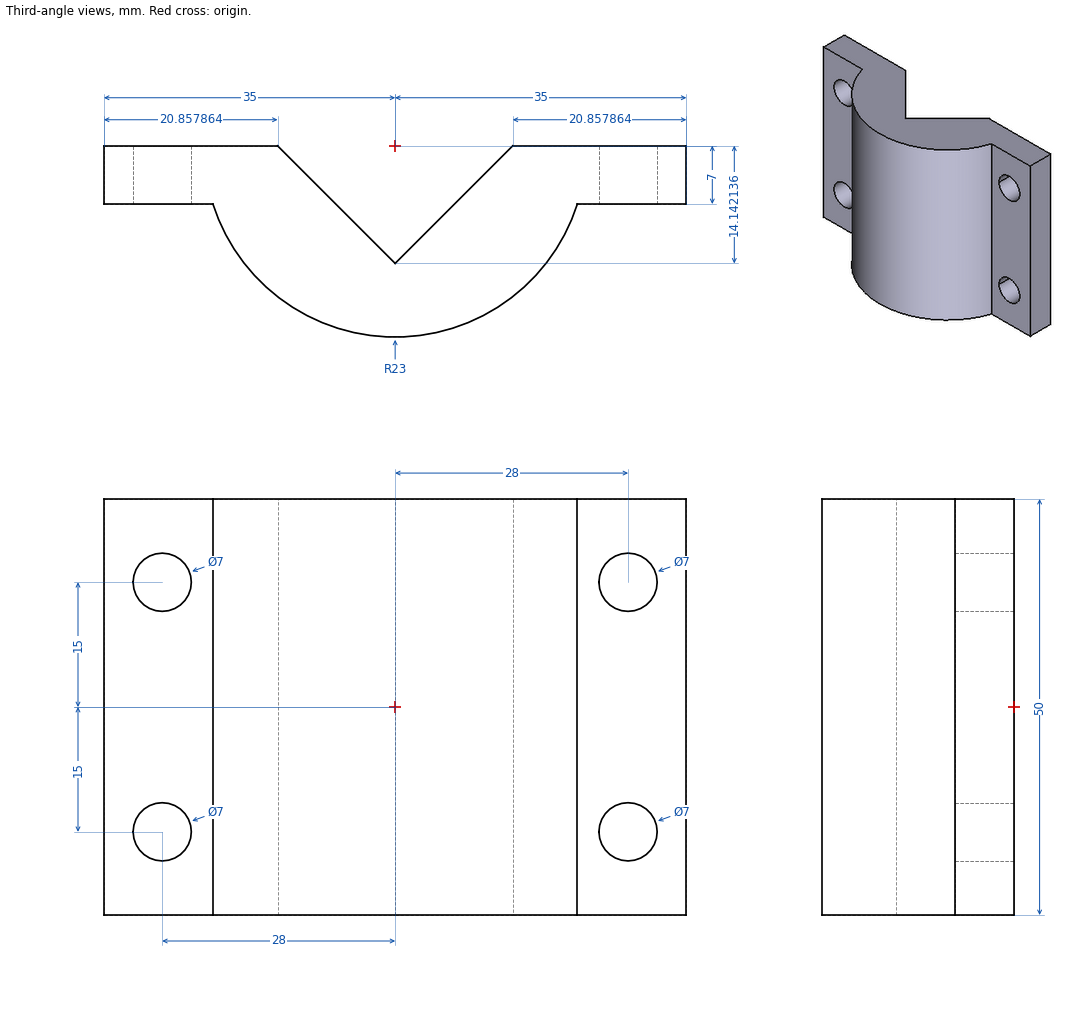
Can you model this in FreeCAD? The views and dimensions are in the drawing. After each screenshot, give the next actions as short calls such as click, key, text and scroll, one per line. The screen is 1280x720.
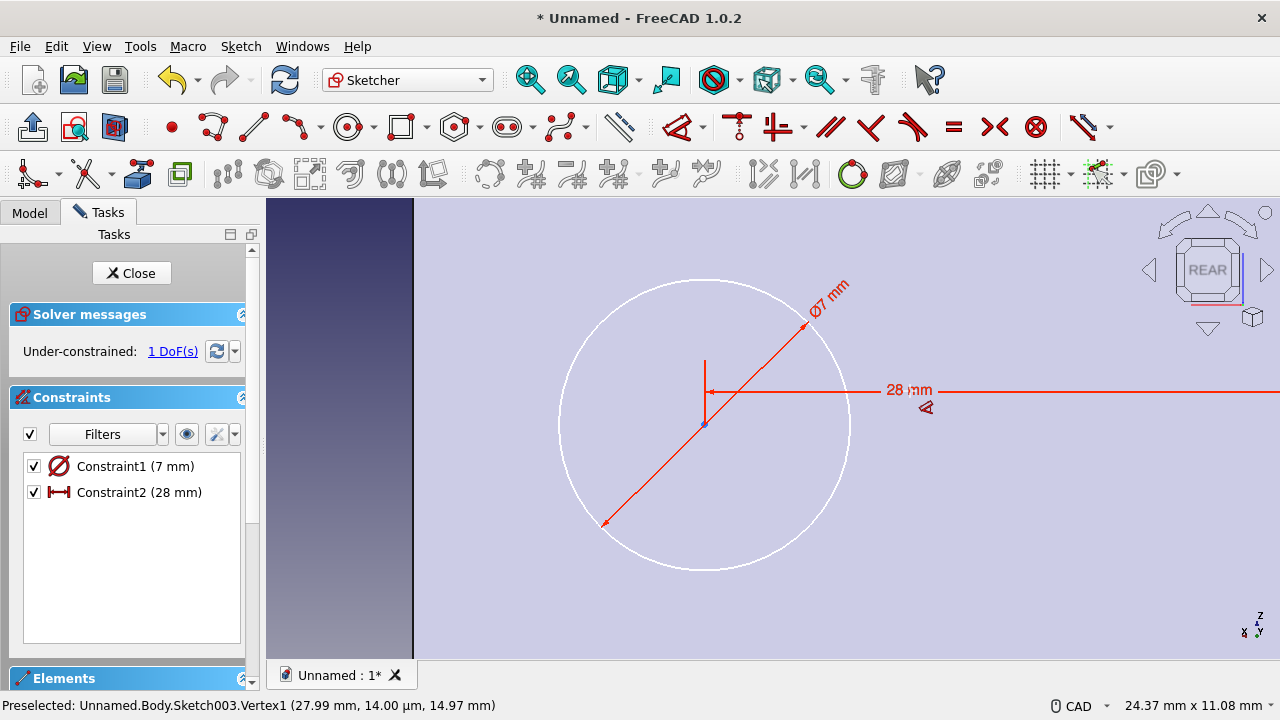
click(705, 425)
click(671, 528)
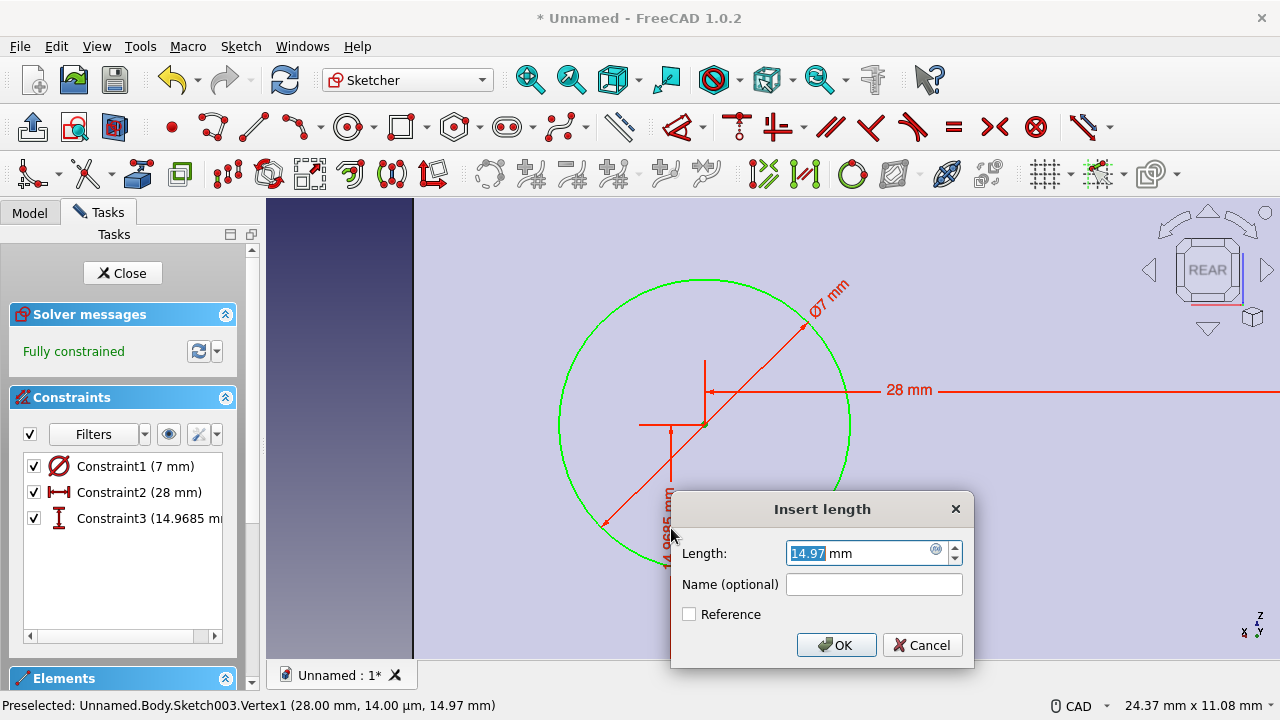
text(15)
key(Return)
key(Escape)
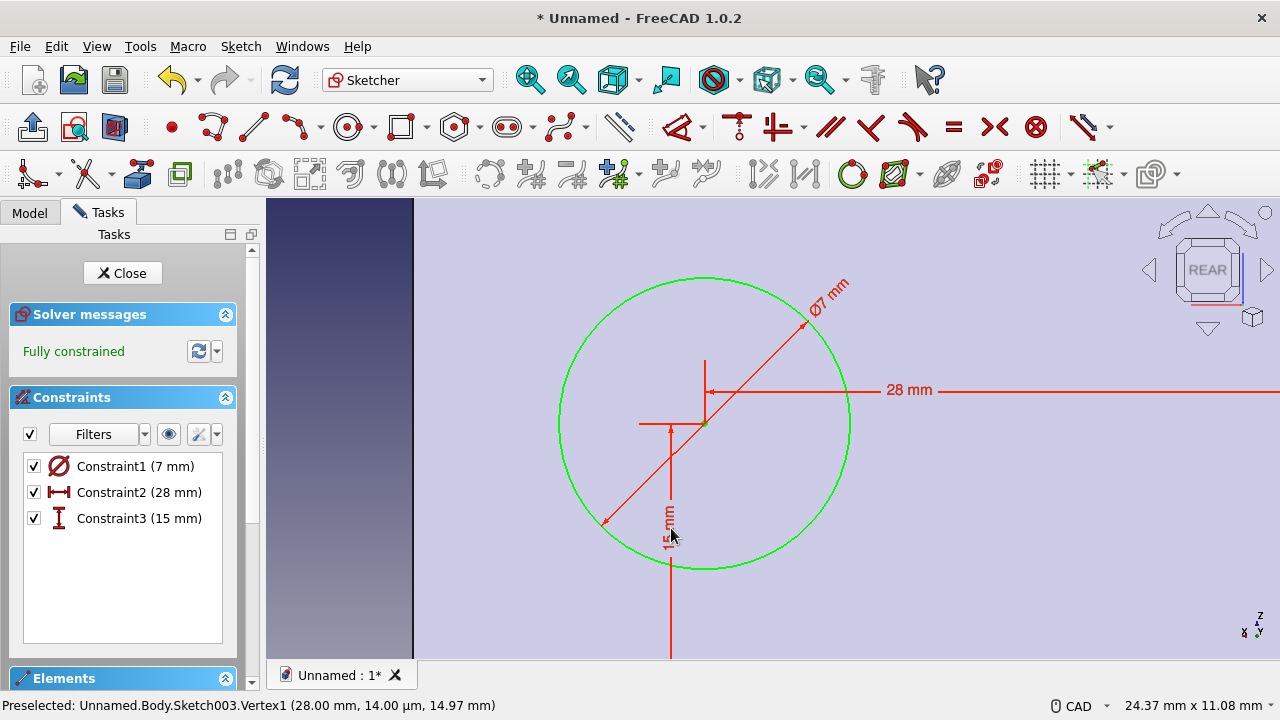
click(123, 273)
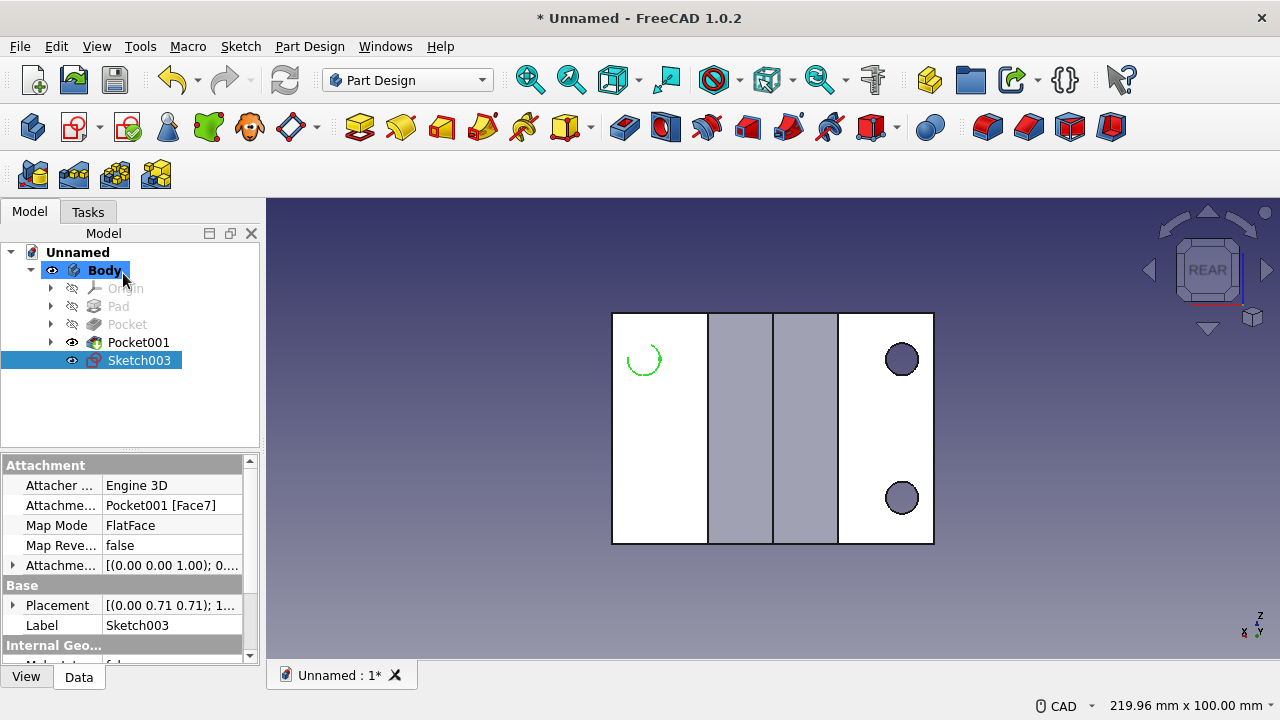
click(625, 128)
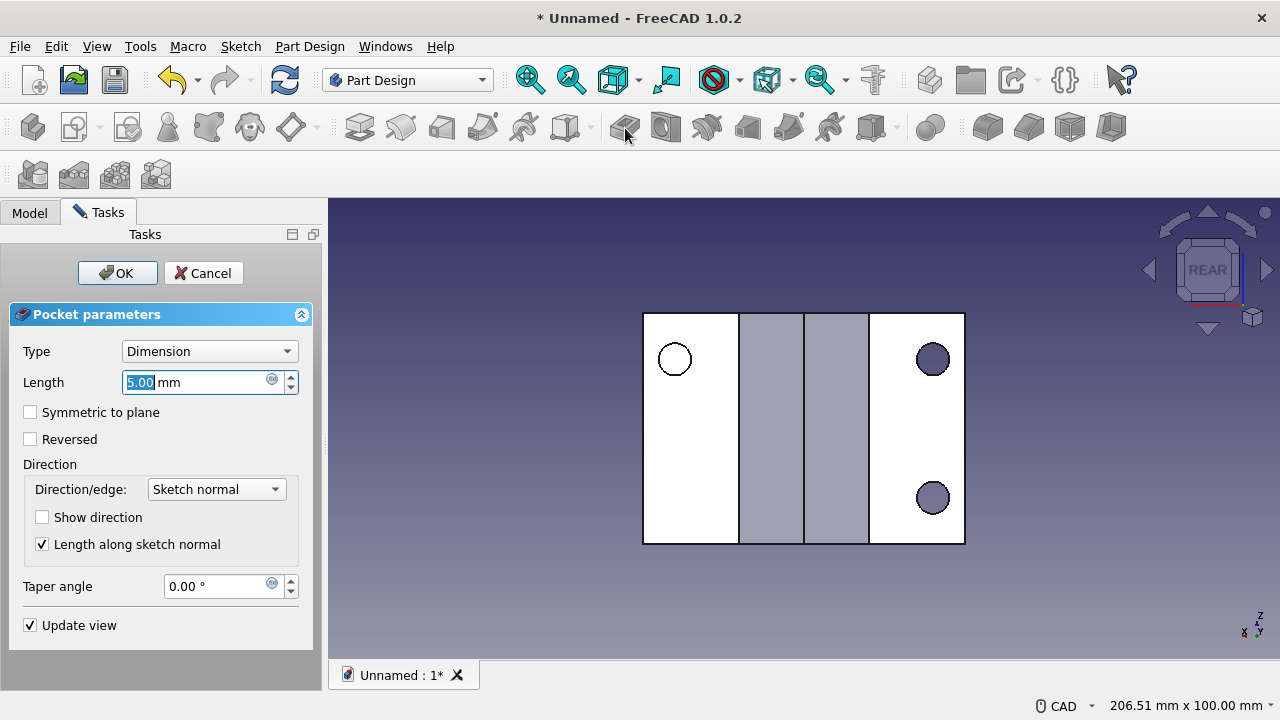
click(210, 352)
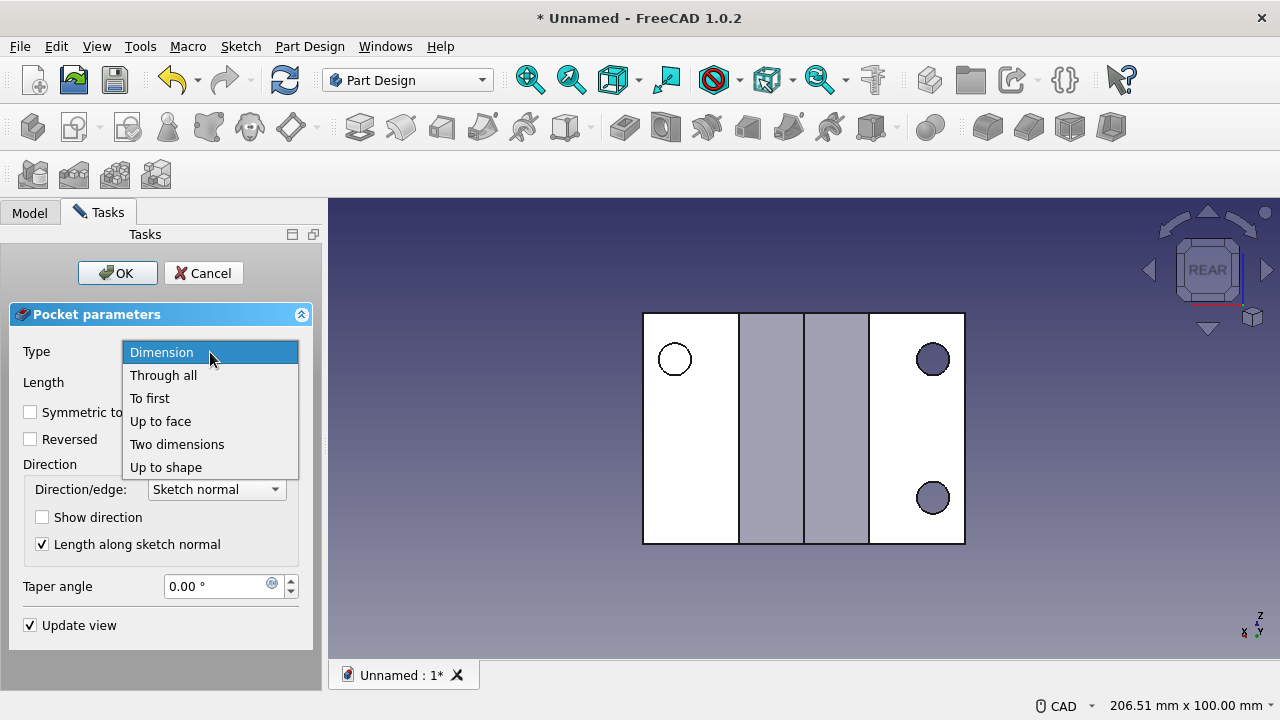
click(208, 398)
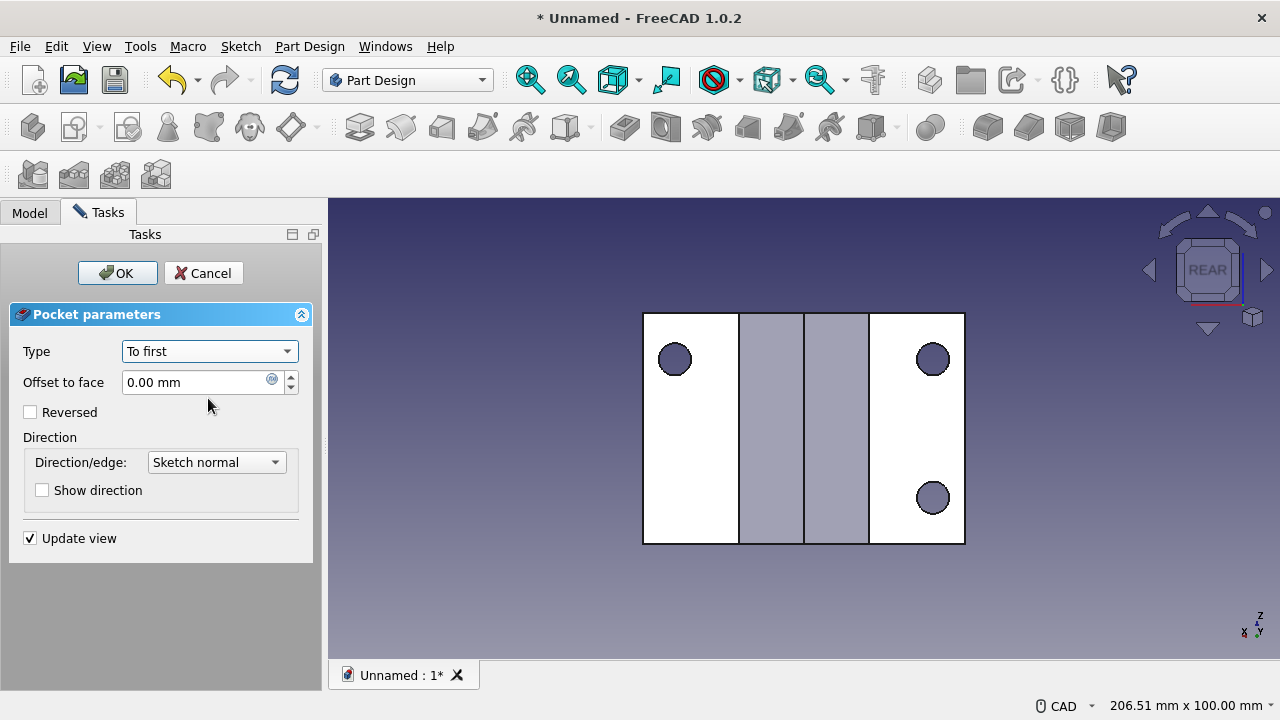
click(118, 273)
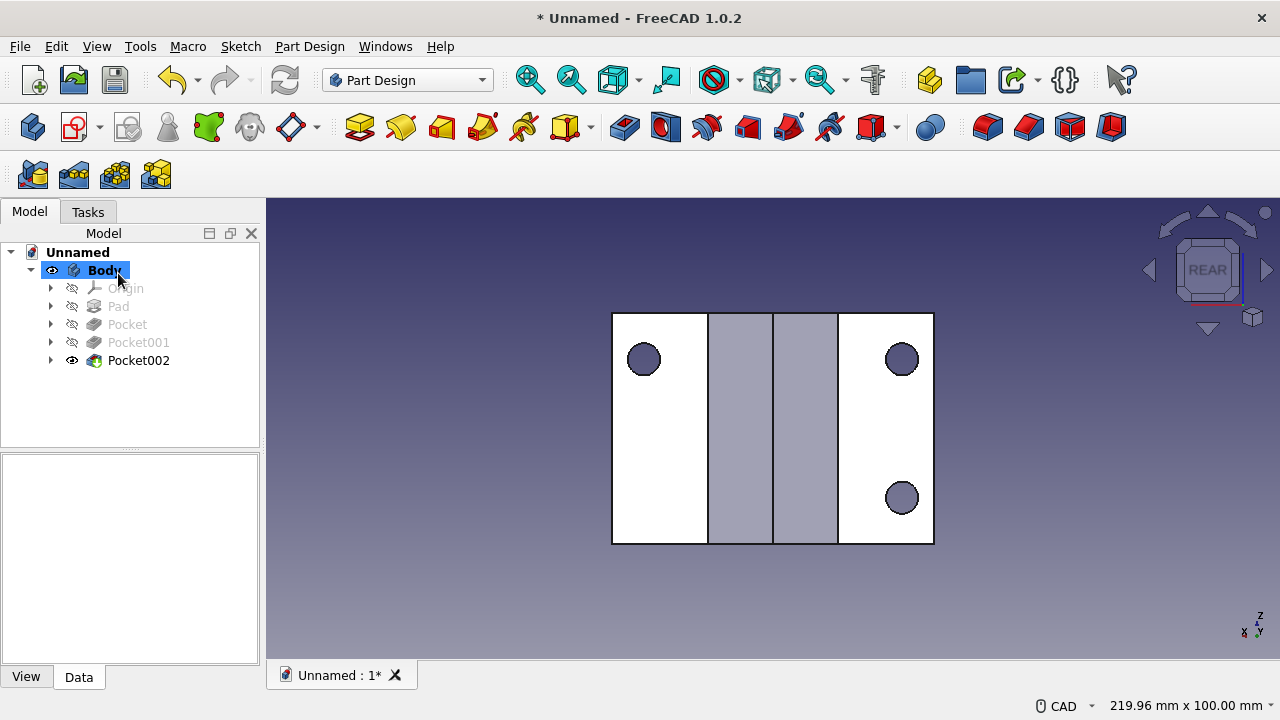
click(660, 427)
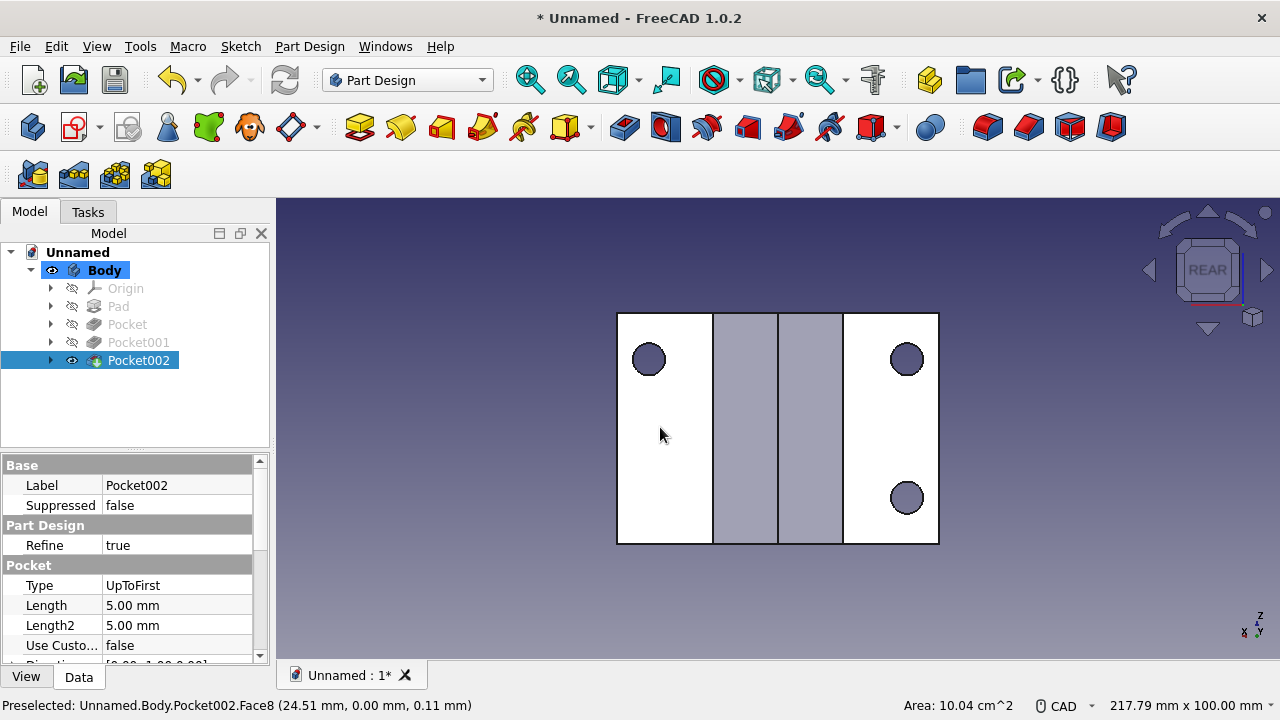
click(74, 128)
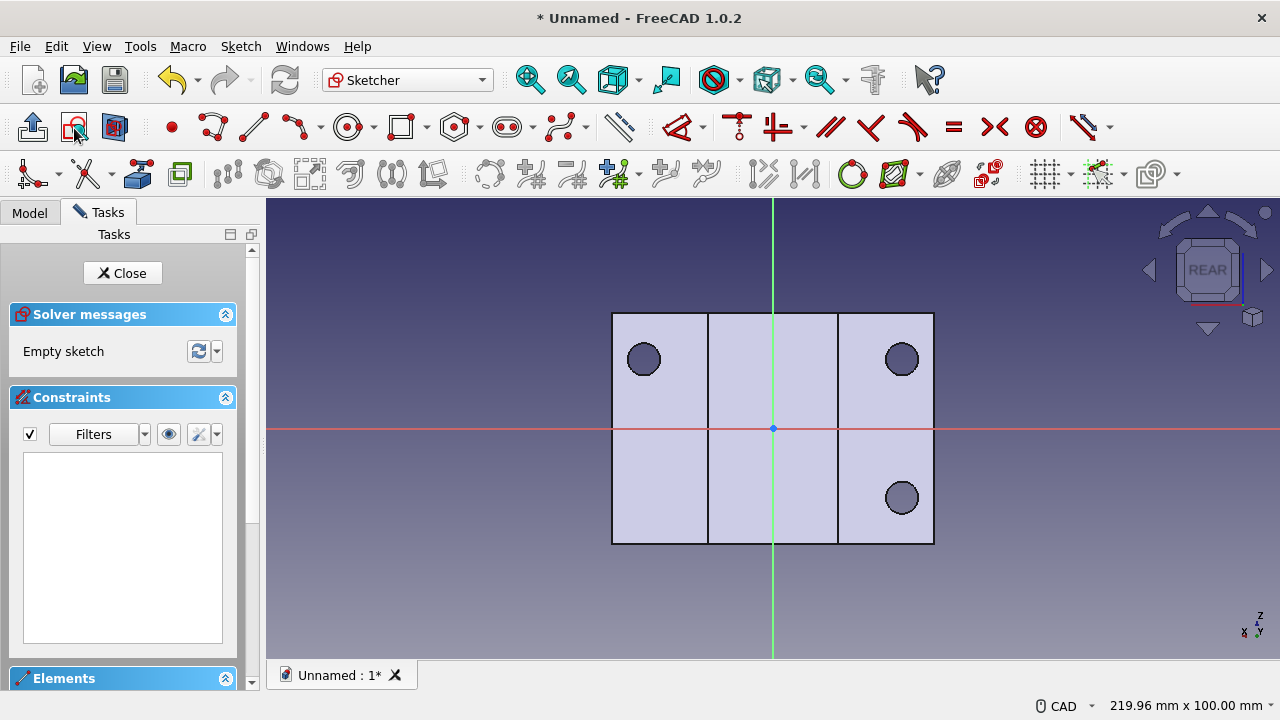
scroll(636, 506, up, 11)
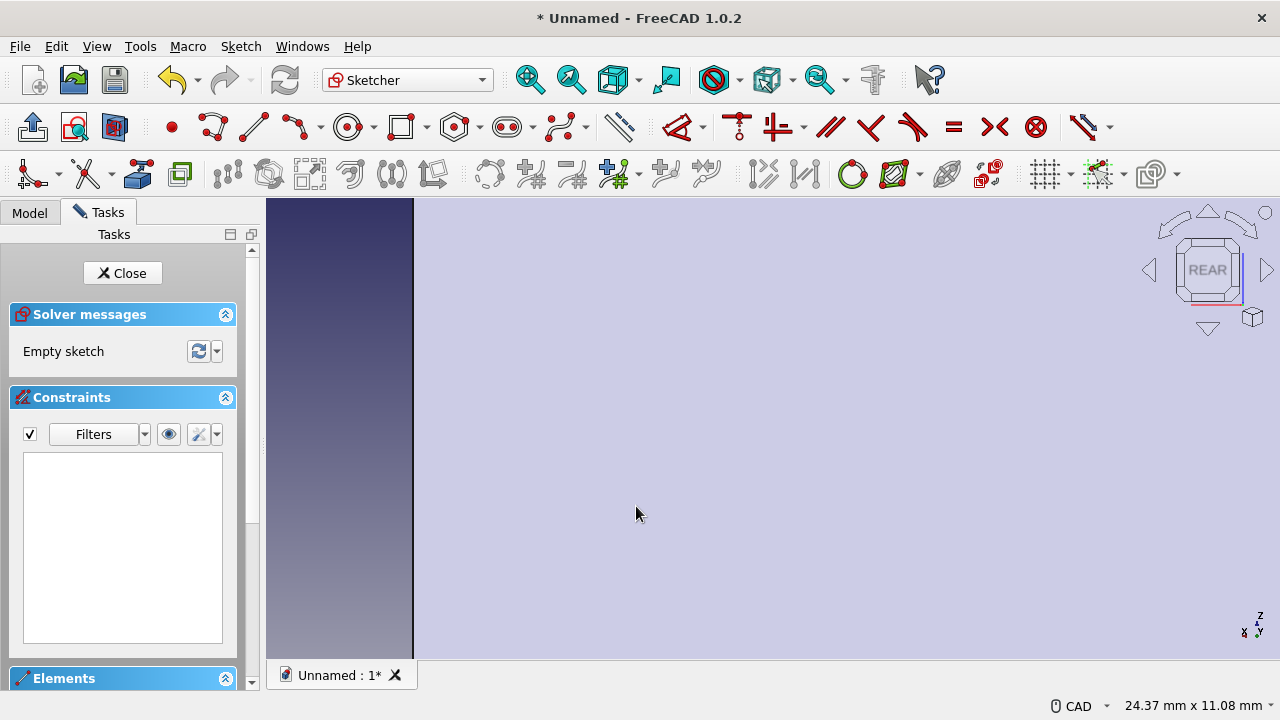
key(g)
key(c)